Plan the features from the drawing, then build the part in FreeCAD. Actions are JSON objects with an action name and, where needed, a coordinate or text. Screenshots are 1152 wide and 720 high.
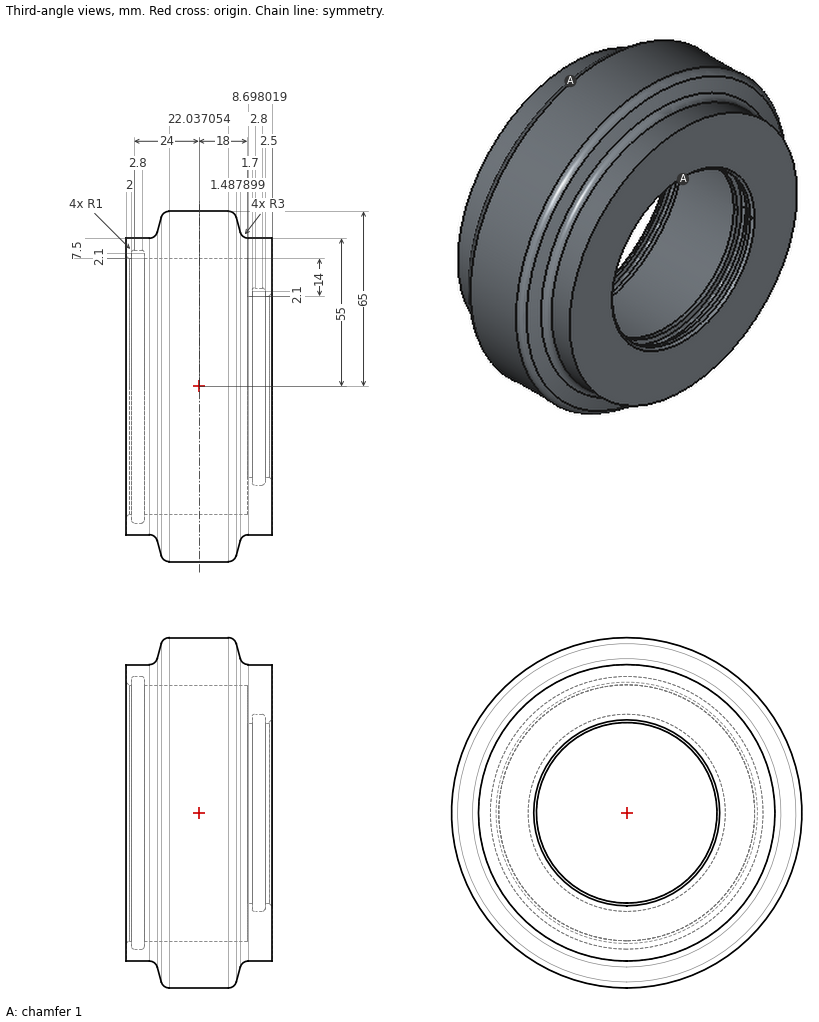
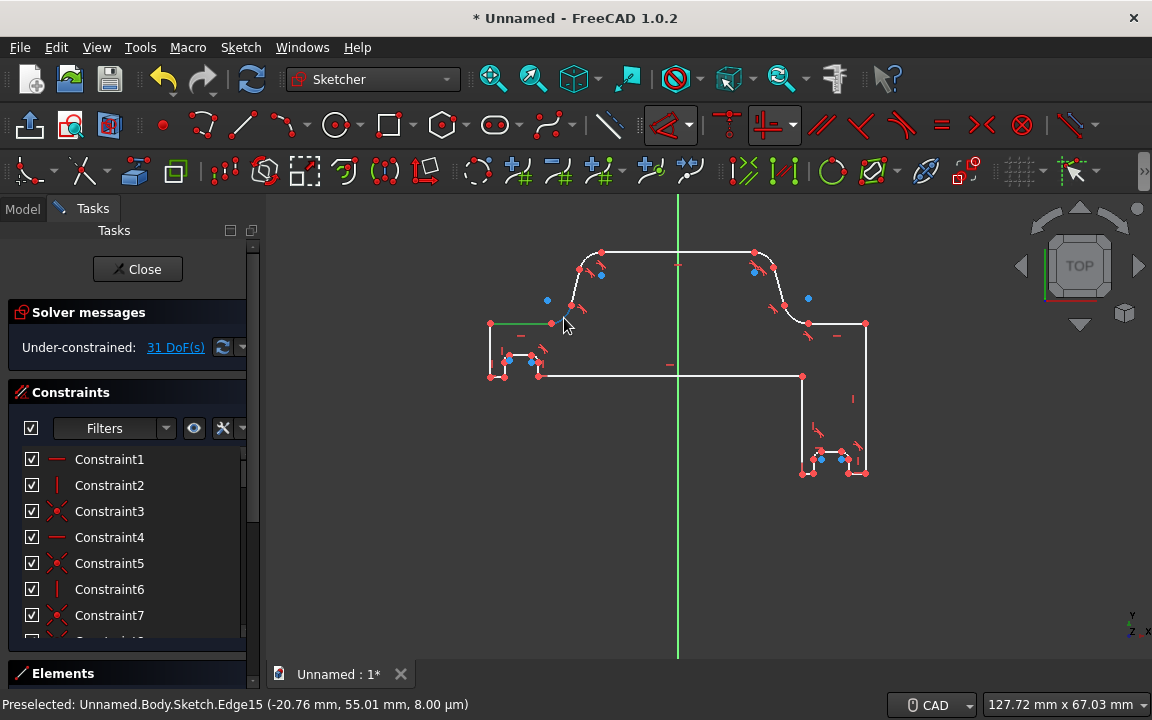
{"action": "left_click", "coordinate": [564, 318]}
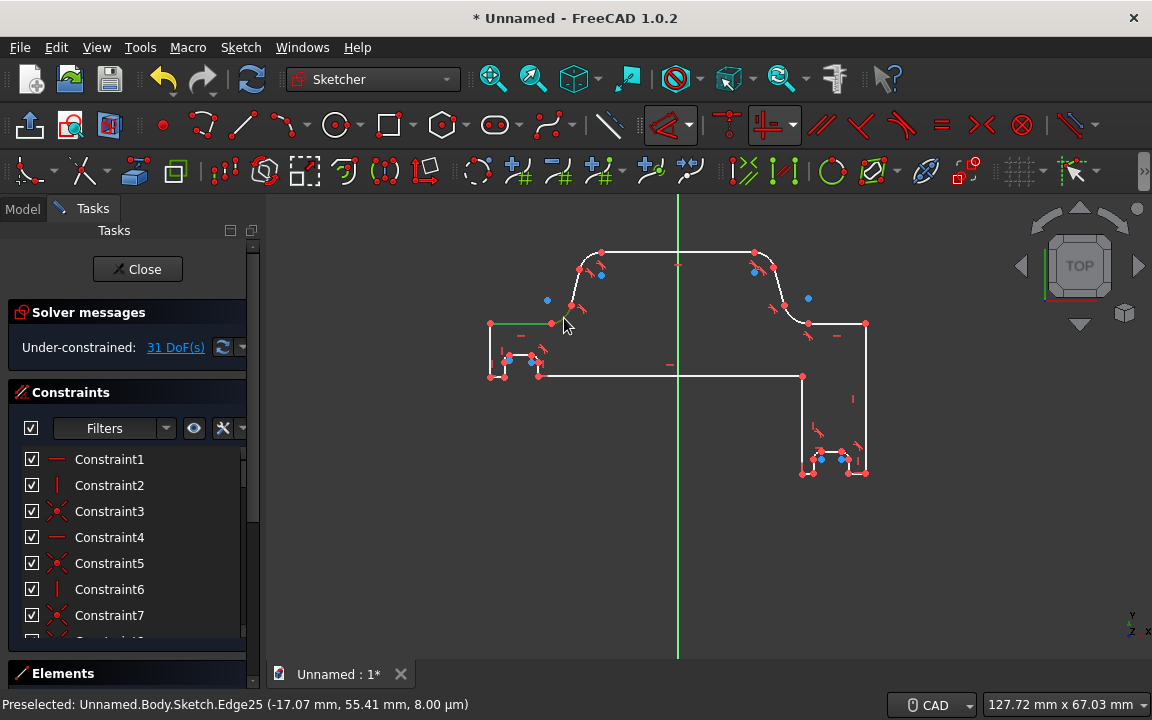
{"action": "key", "text": "t"}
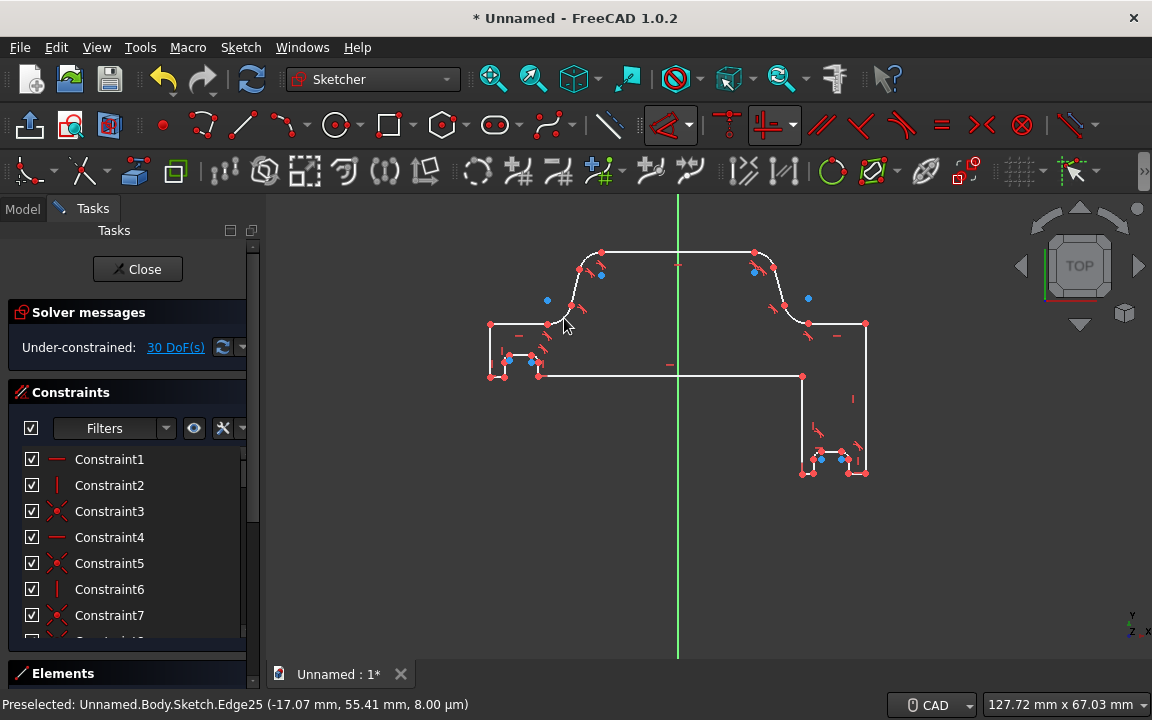
{"action": "scroll", "coordinate": [505, 370], "scroll_direction": "up", "scroll_amount": 3}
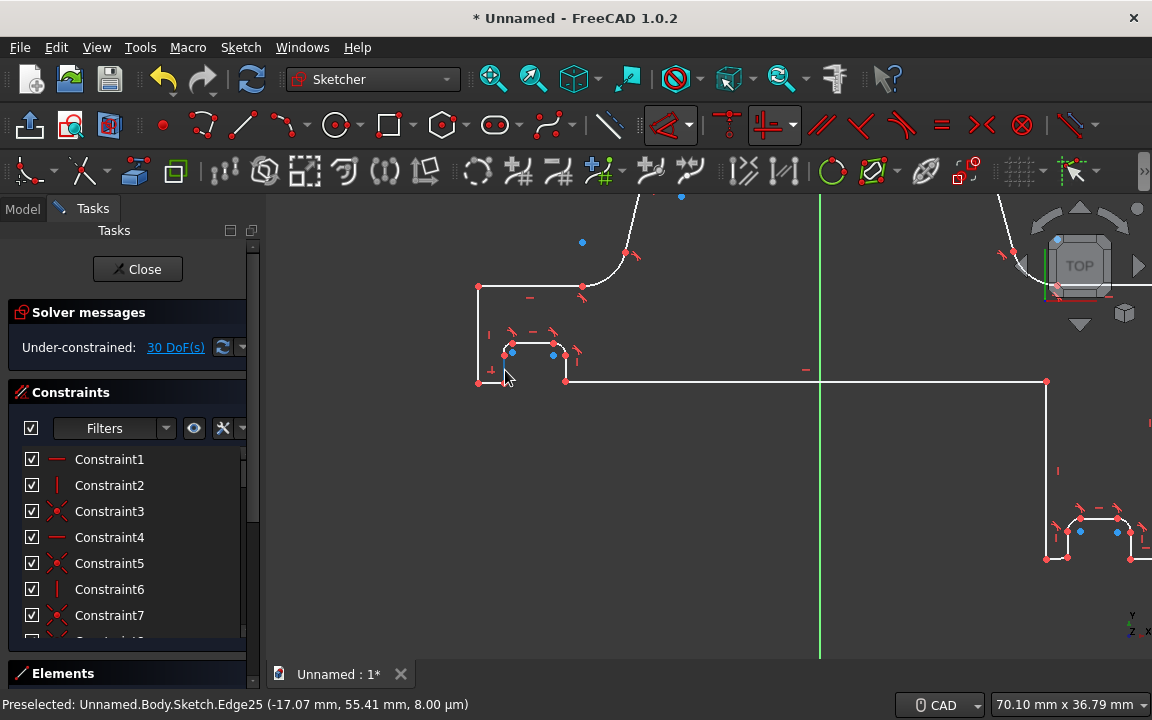
{"action": "left_click", "coordinate": [504, 369]}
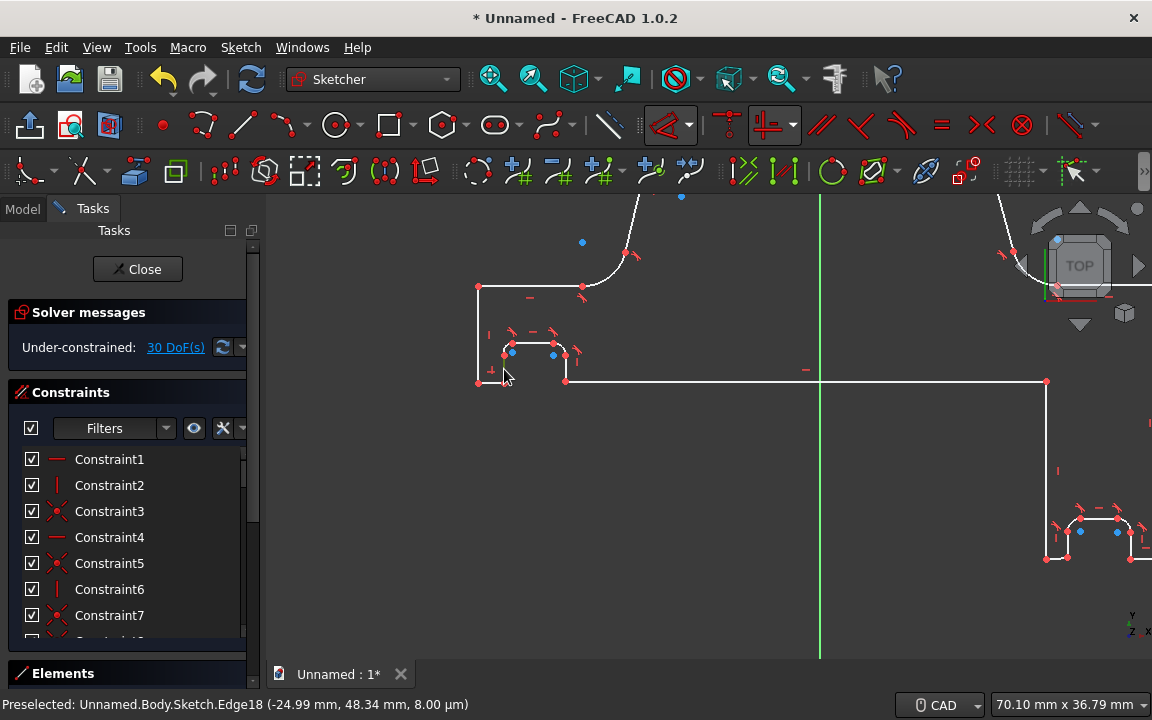
{"action": "scroll", "coordinate": [505, 347], "scroll_direction": "up", "scroll_amount": 3}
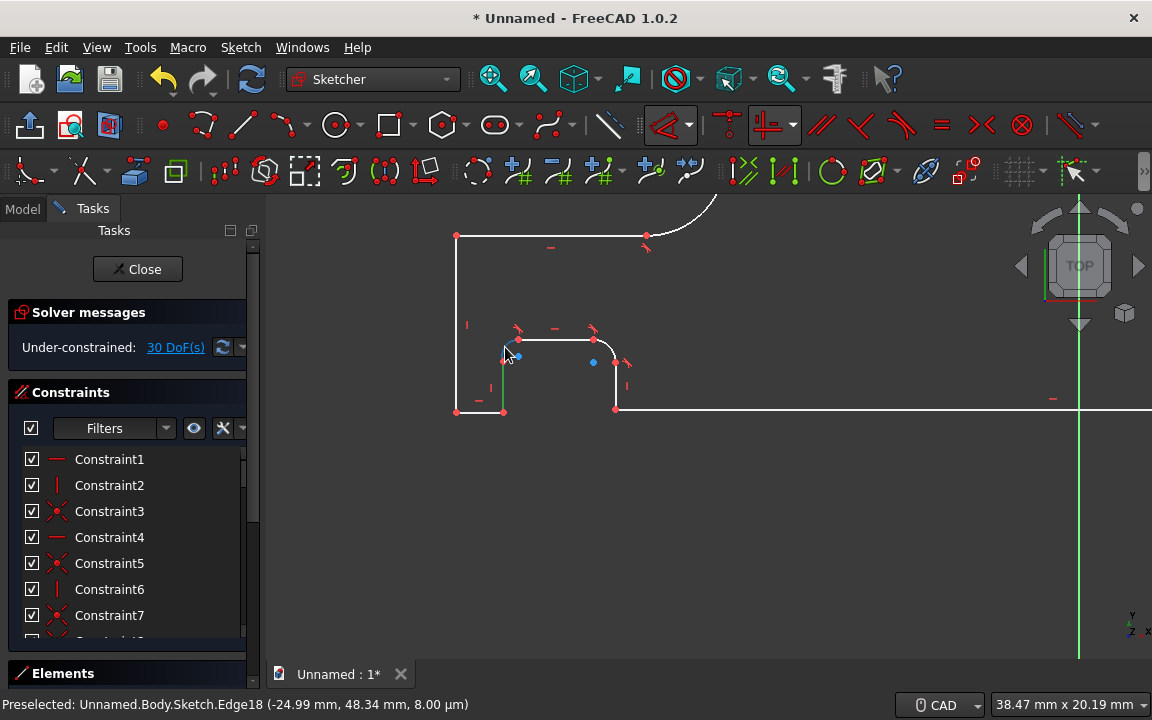
{"action": "left_click", "coordinate": [505, 347]}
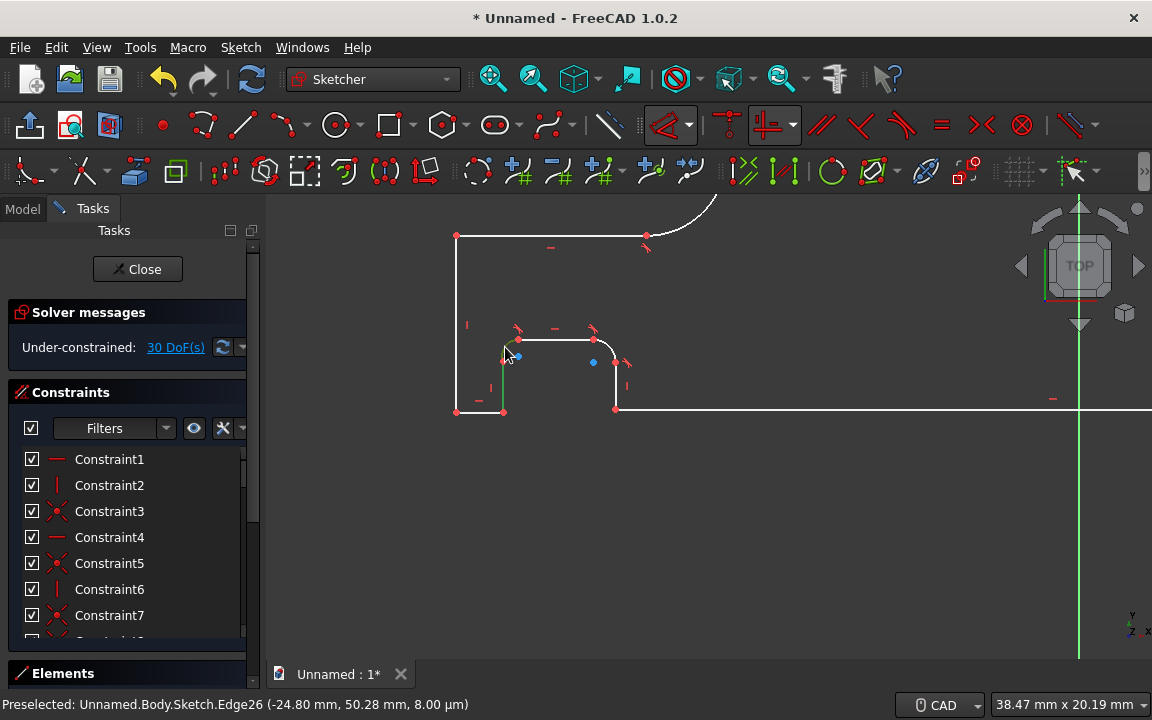
{"action": "left_click", "coordinate": [902, 126]}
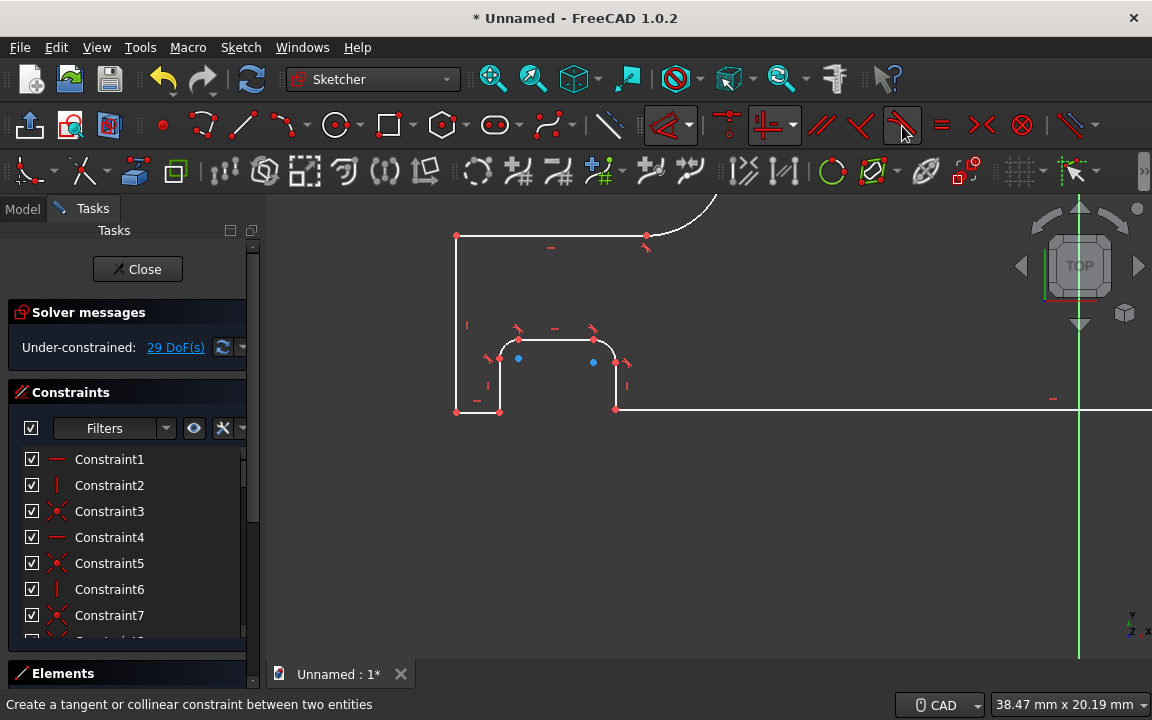
{"action": "scroll", "coordinate": [530, 344], "scroll_direction": "down", "scroll_amount": 8}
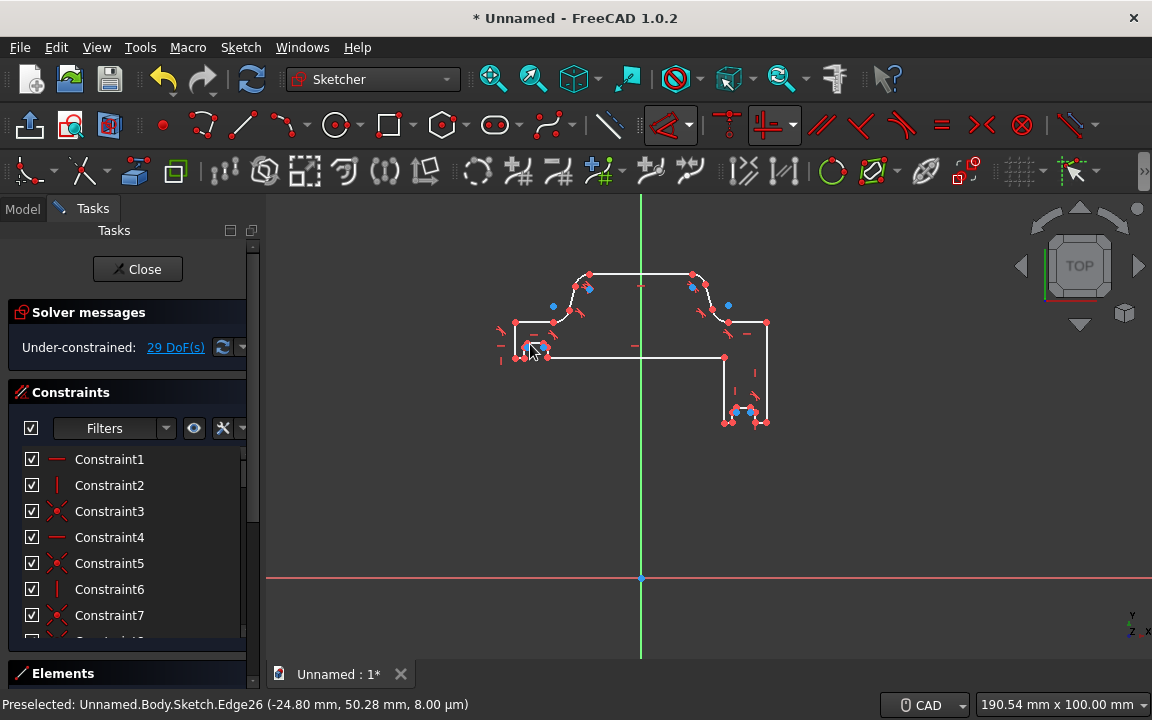
{"action": "scroll", "coordinate": [727, 423], "scroll_direction": "up", "scroll_amount": 9}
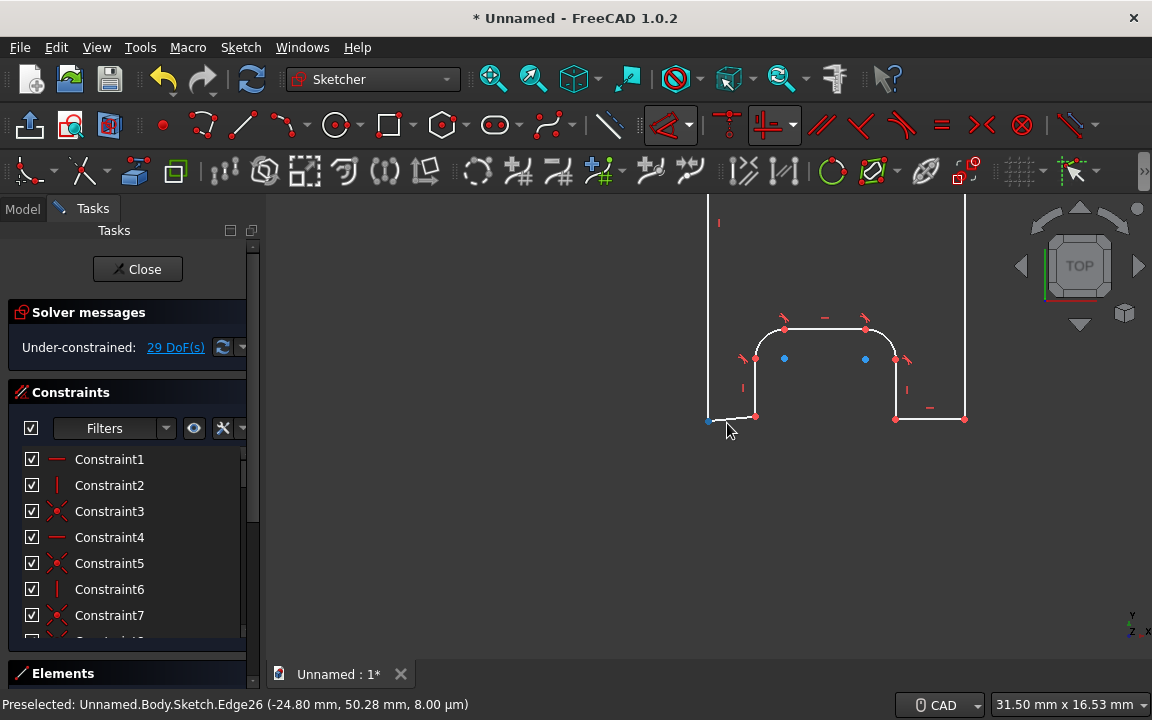
{"action": "left_click", "coordinate": [722, 420]}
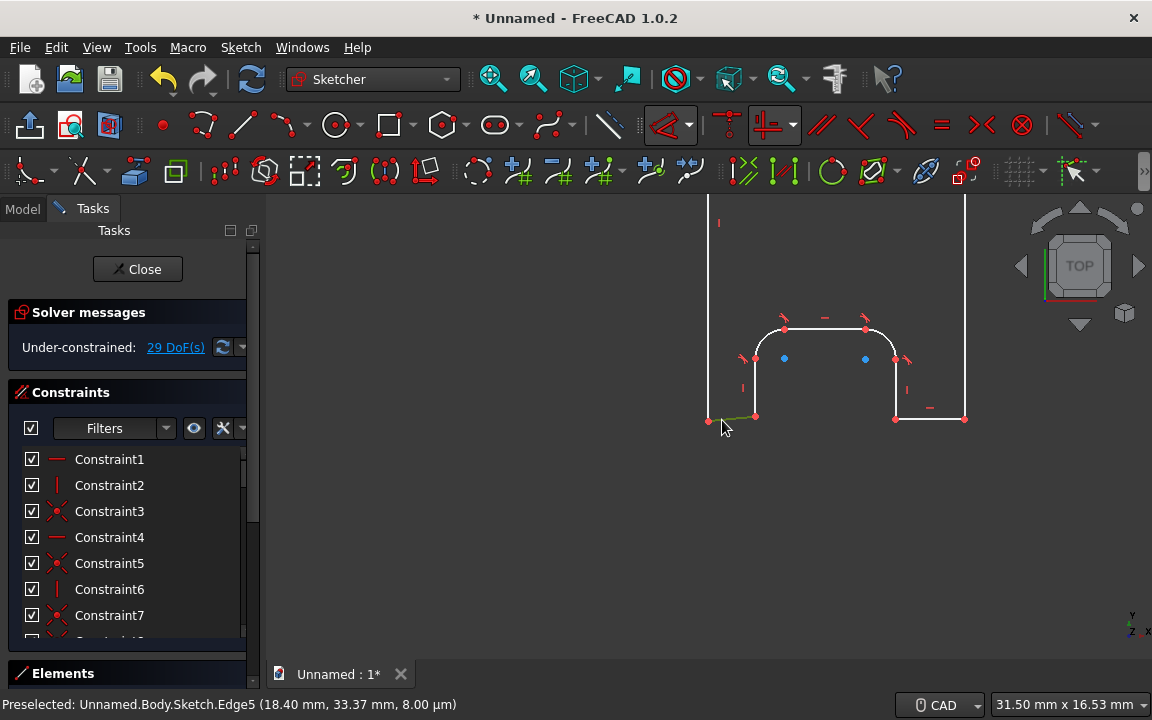
{"action": "key", "text": "h"}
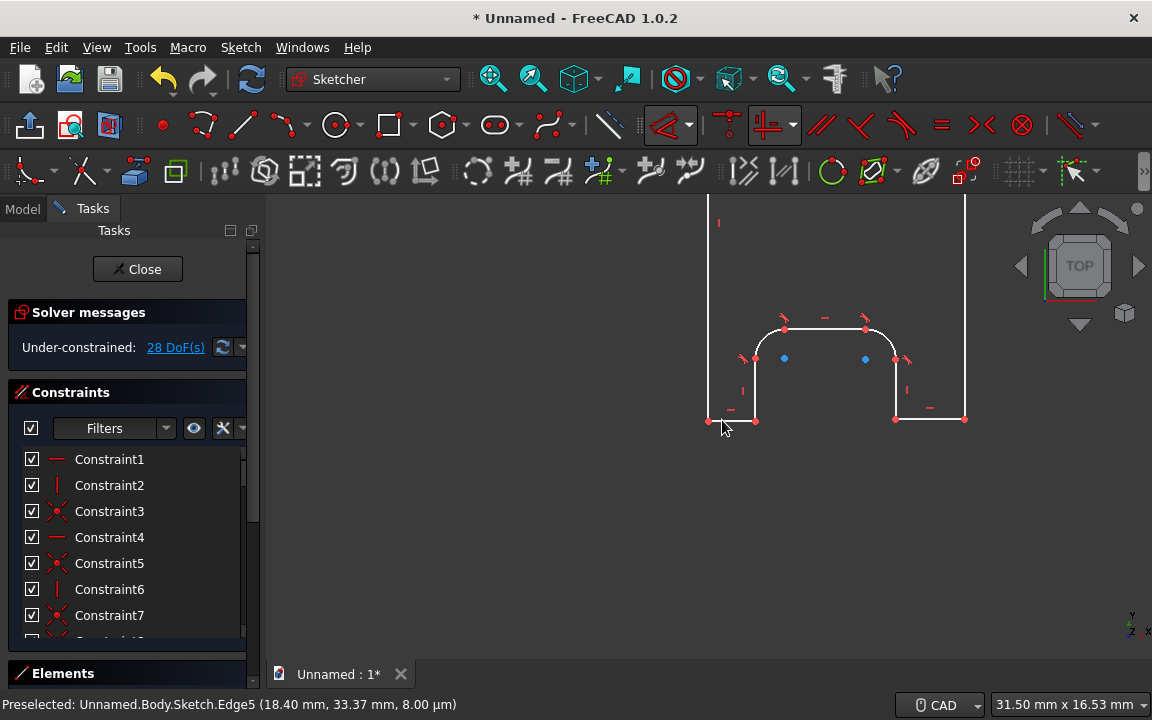
{"action": "scroll", "coordinate": [727, 423], "scroll_direction": "down", "scroll_amount": 9}